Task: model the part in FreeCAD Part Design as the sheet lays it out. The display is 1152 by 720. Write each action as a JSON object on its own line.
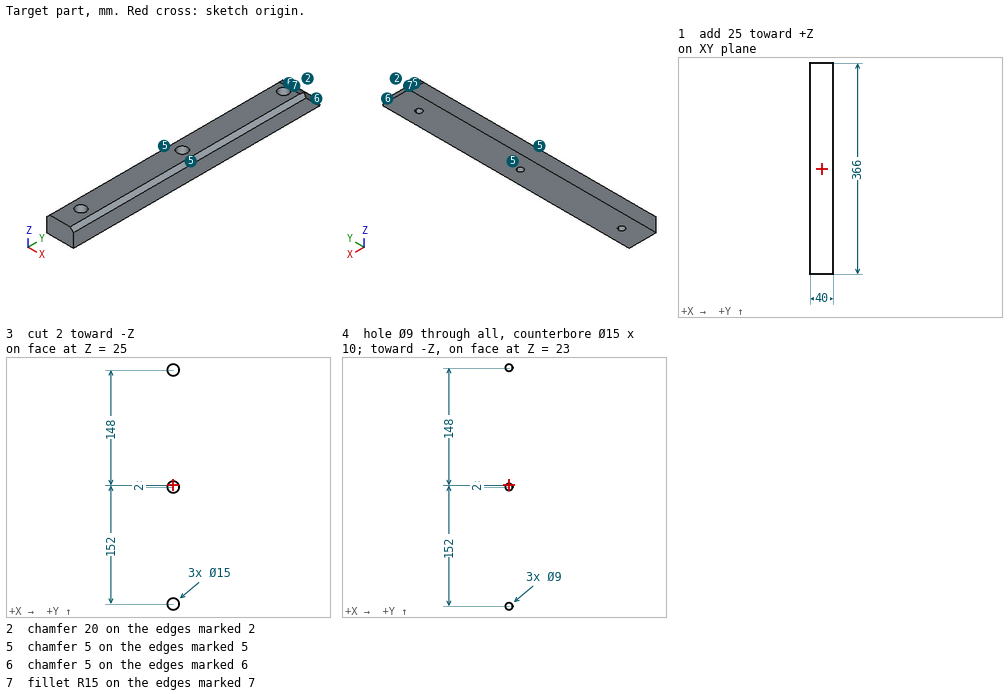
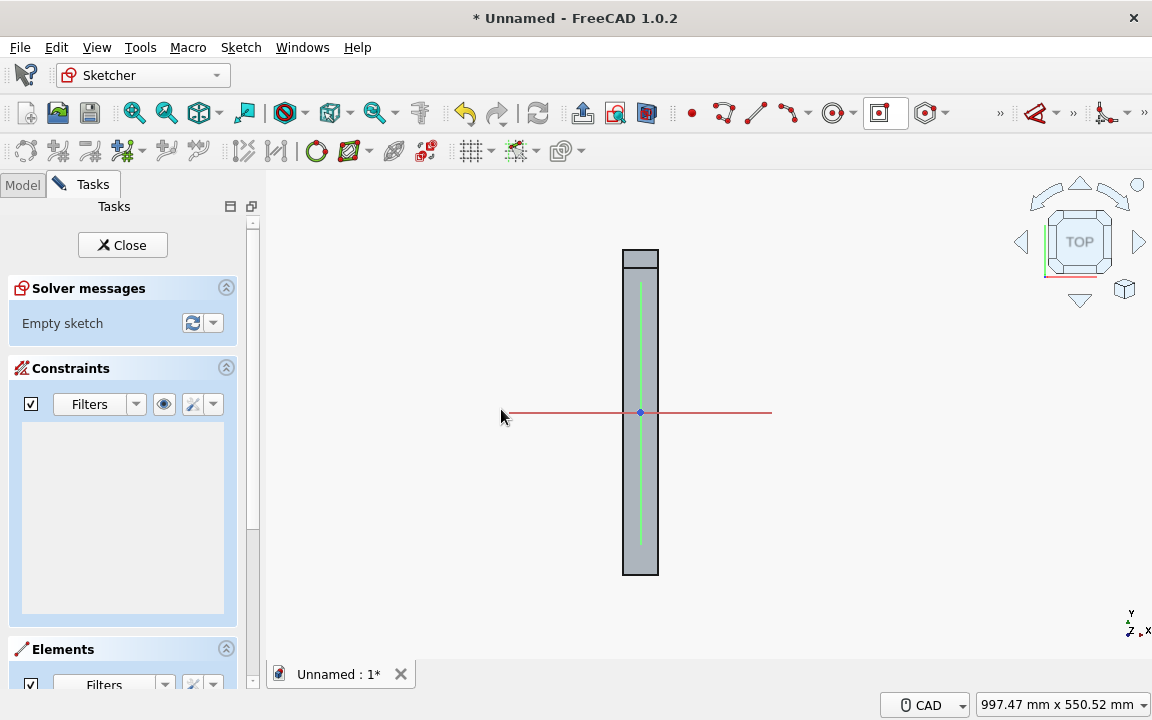
{"action": "left_click", "coordinate": [834, 114]}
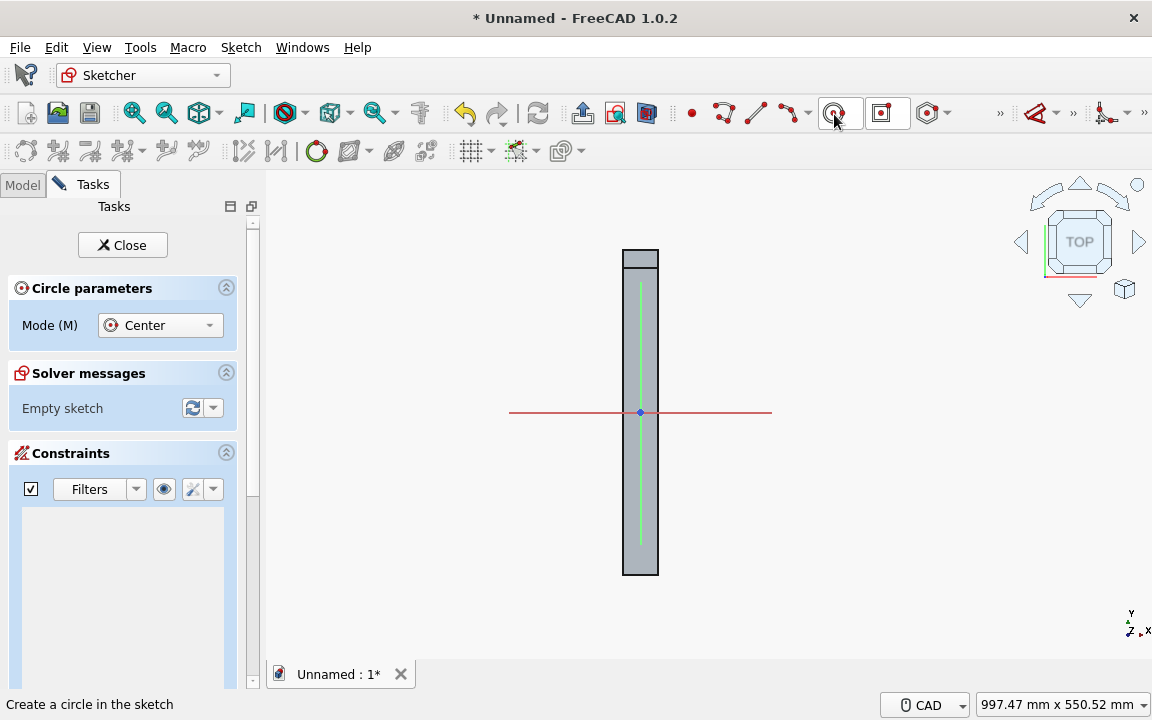
{"action": "scroll", "coordinate": [641, 548], "scroll_direction": "up", "scroll_amount": 7}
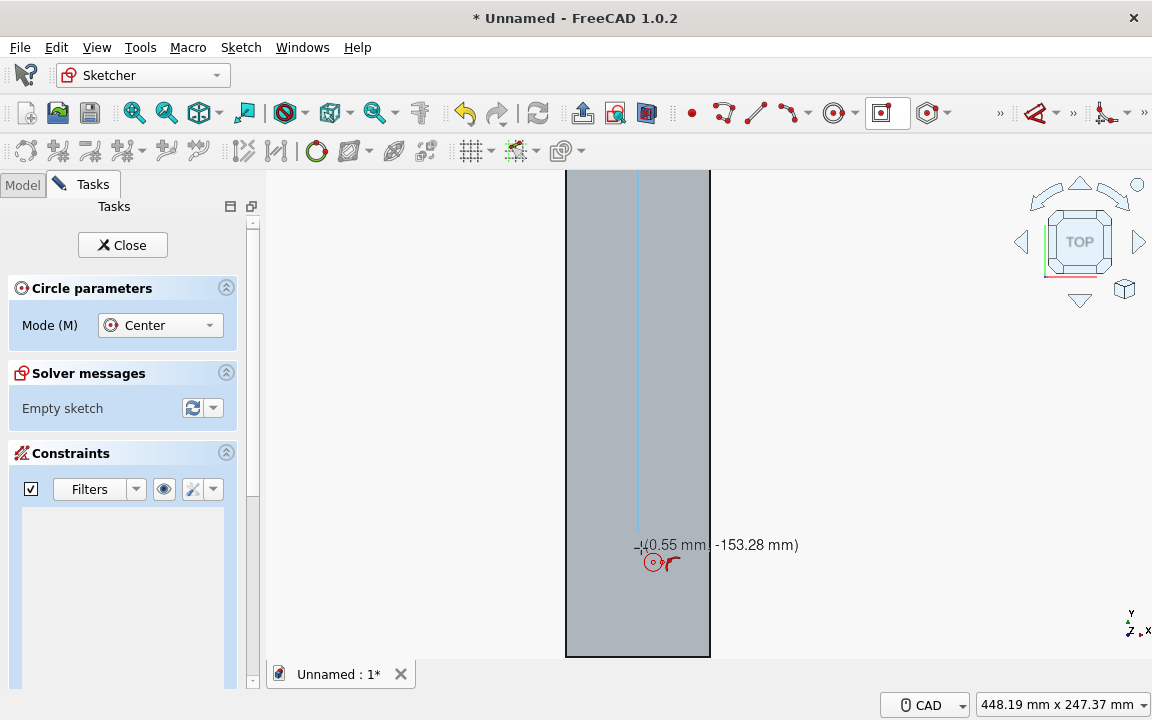
{"action": "scroll", "coordinate": [641, 549], "scroll_direction": "down", "scroll_amount": 7}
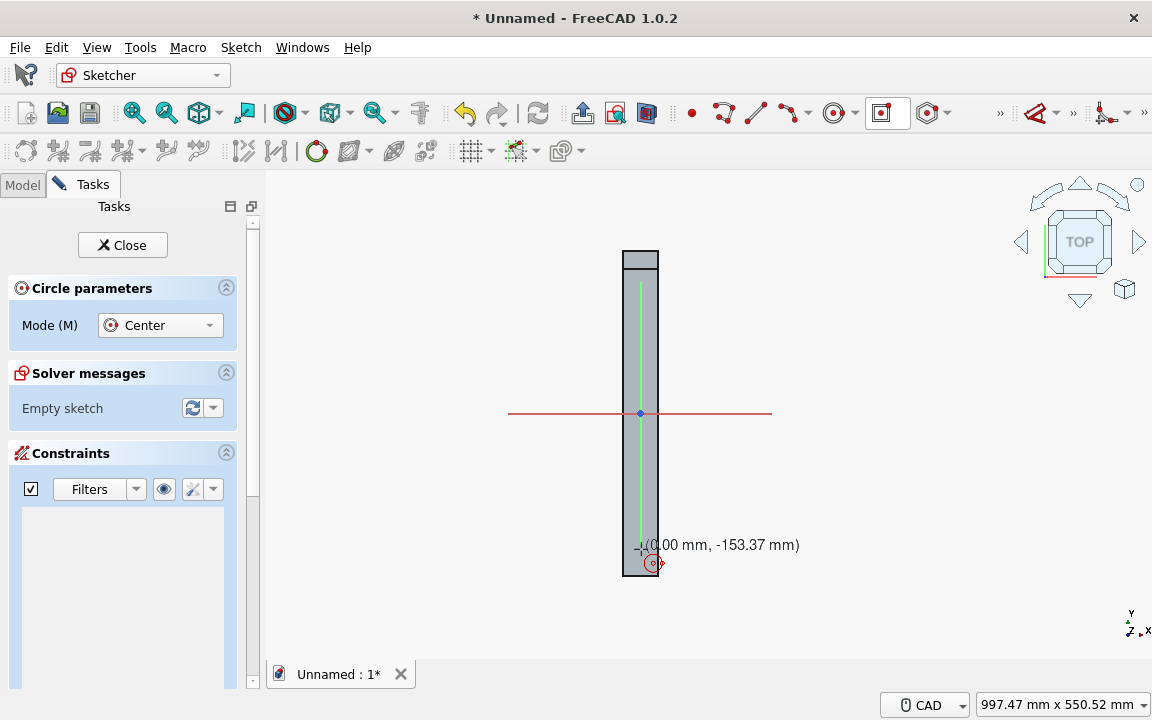
{"action": "left_click", "coordinate": [641, 549]}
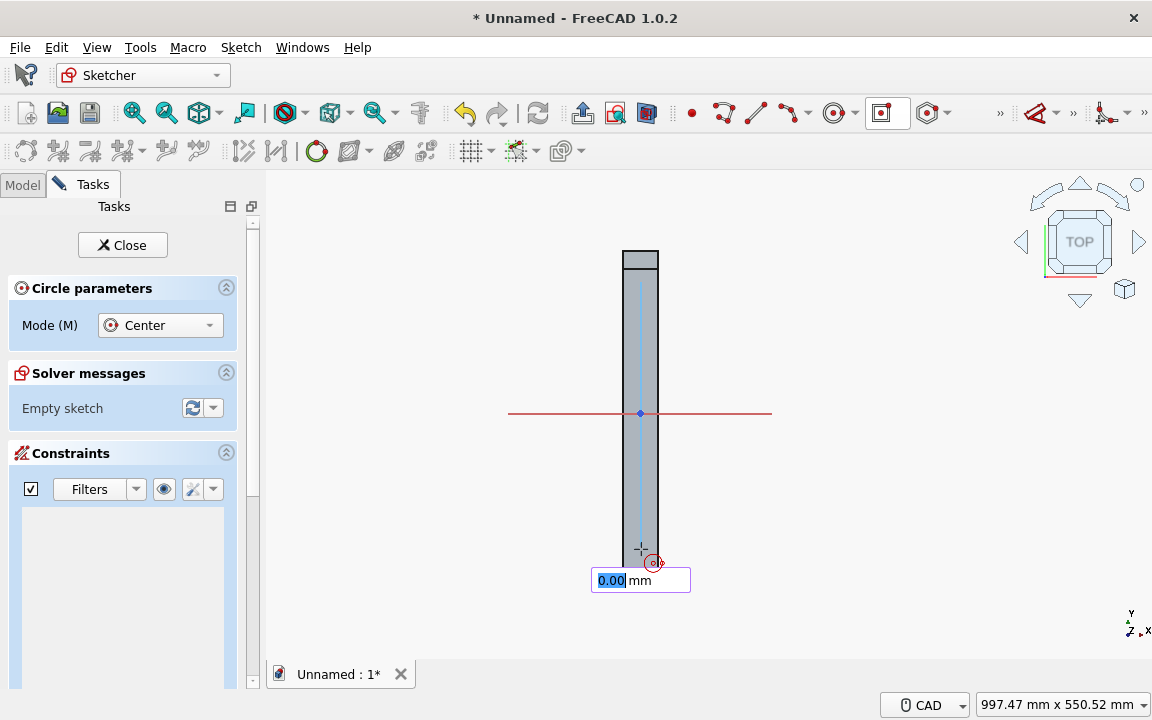
{"action": "scroll", "coordinate": [647, 546], "scroll_direction": "up", "scroll_amount": 5}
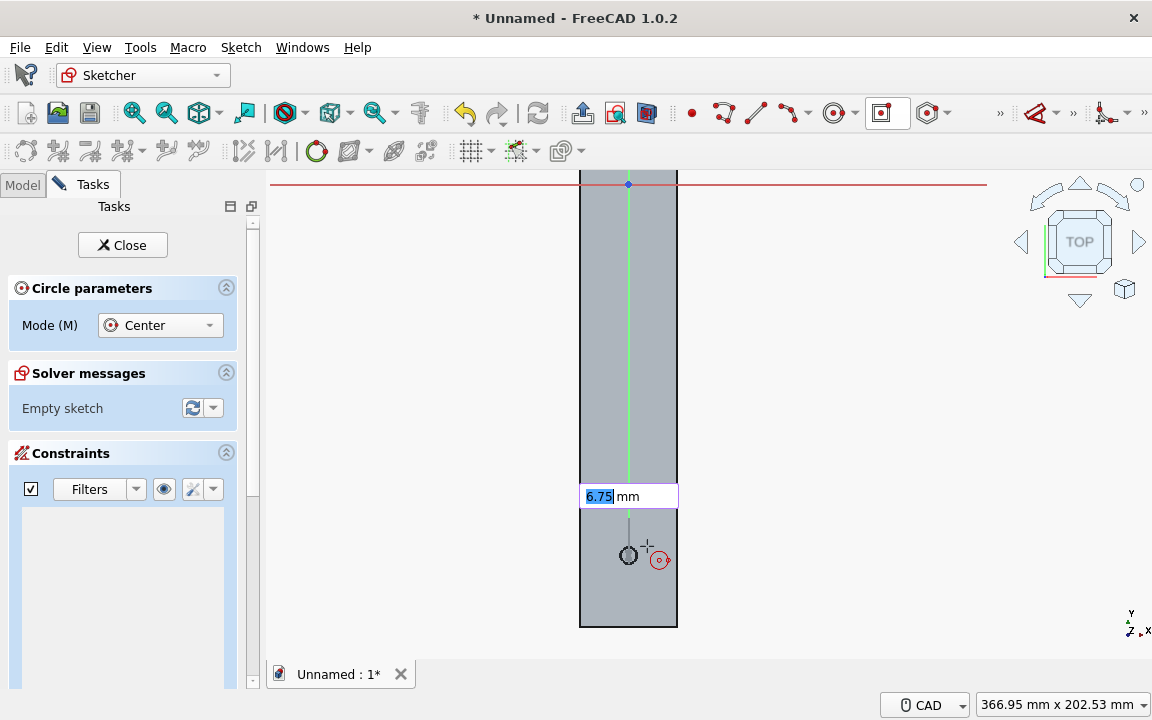
{"action": "left_click", "coordinate": [646, 546]}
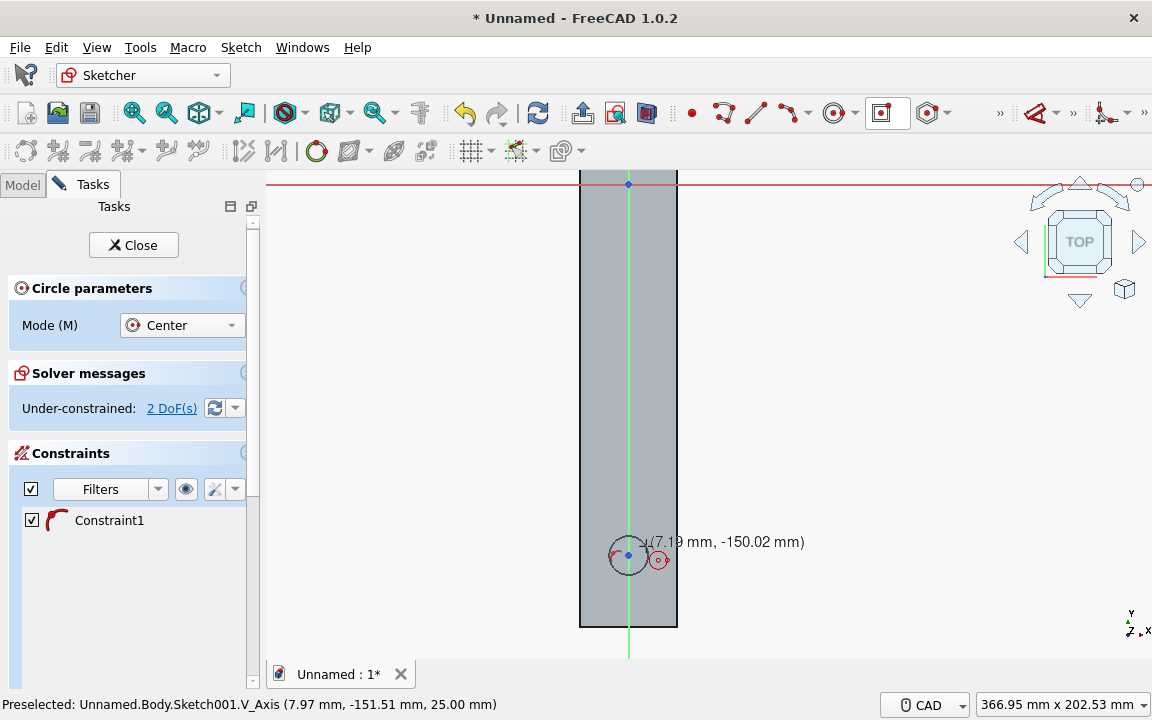
{"action": "scroll", "coordinate": [647, 545], "scroll_direction": "down", "scroll_amount": 5}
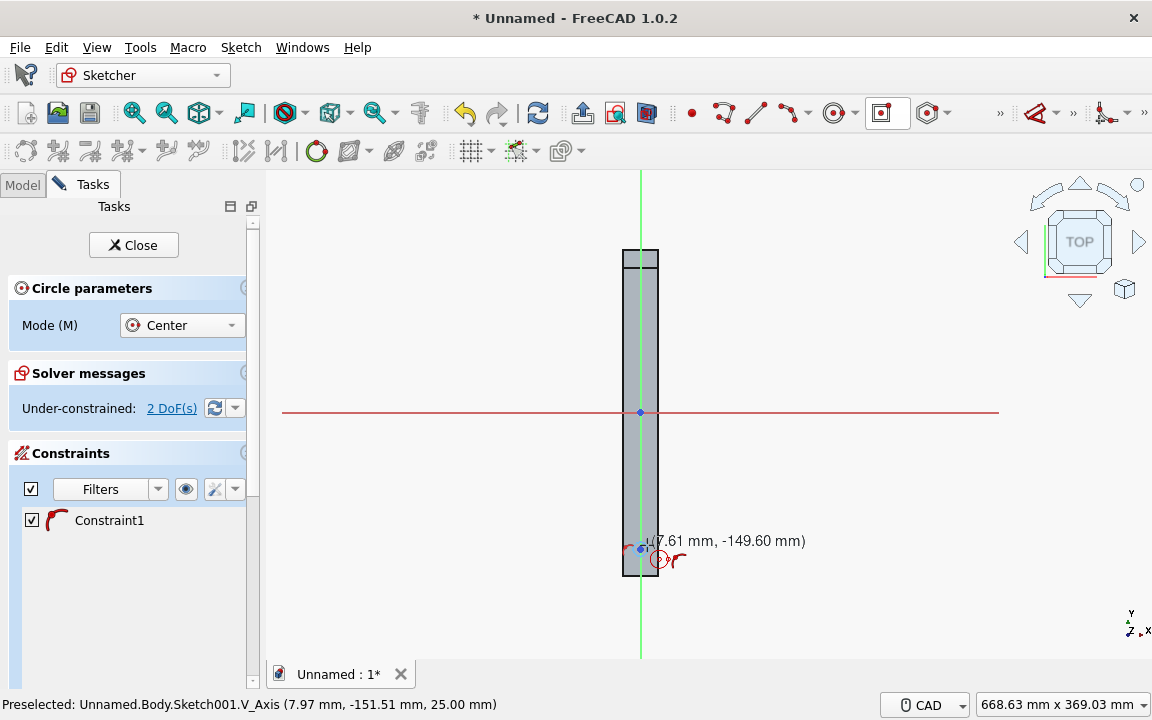
{"action": "scroll", "coordinate": [641, 415], "scroll_direction": "up", "scroll_amount": 11}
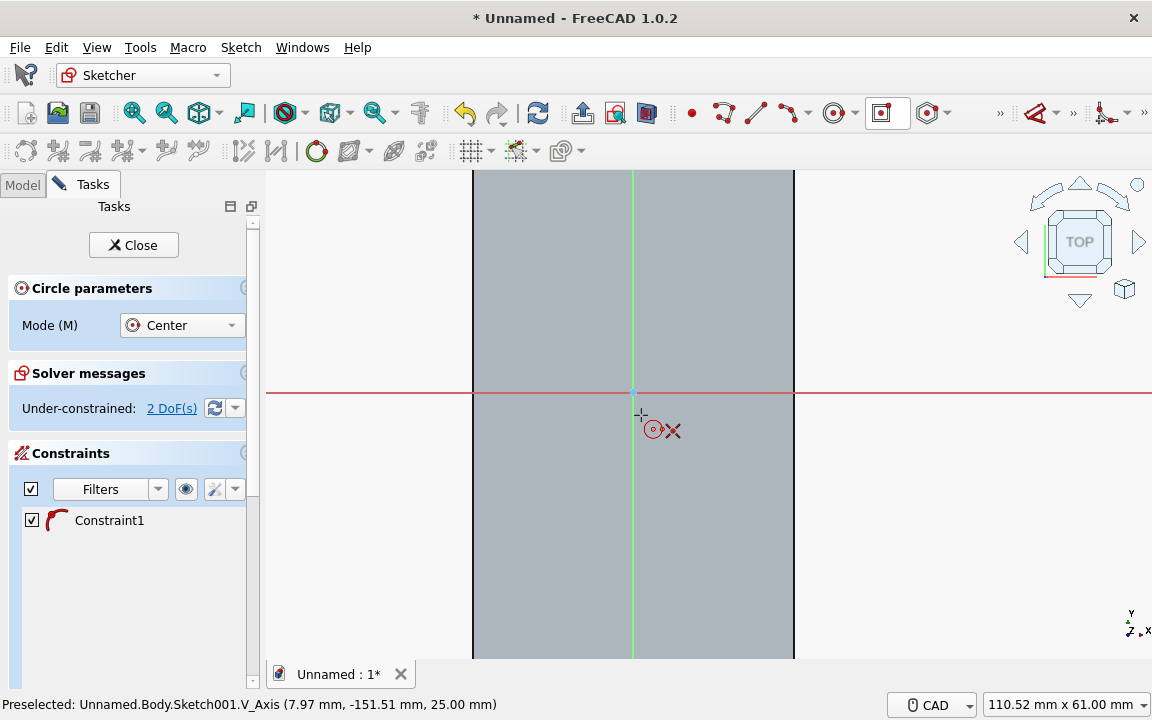
{"action": "left_click", "coordinate": [633, 409]}
{"action": "left_click", "coordinate": [676, 366]}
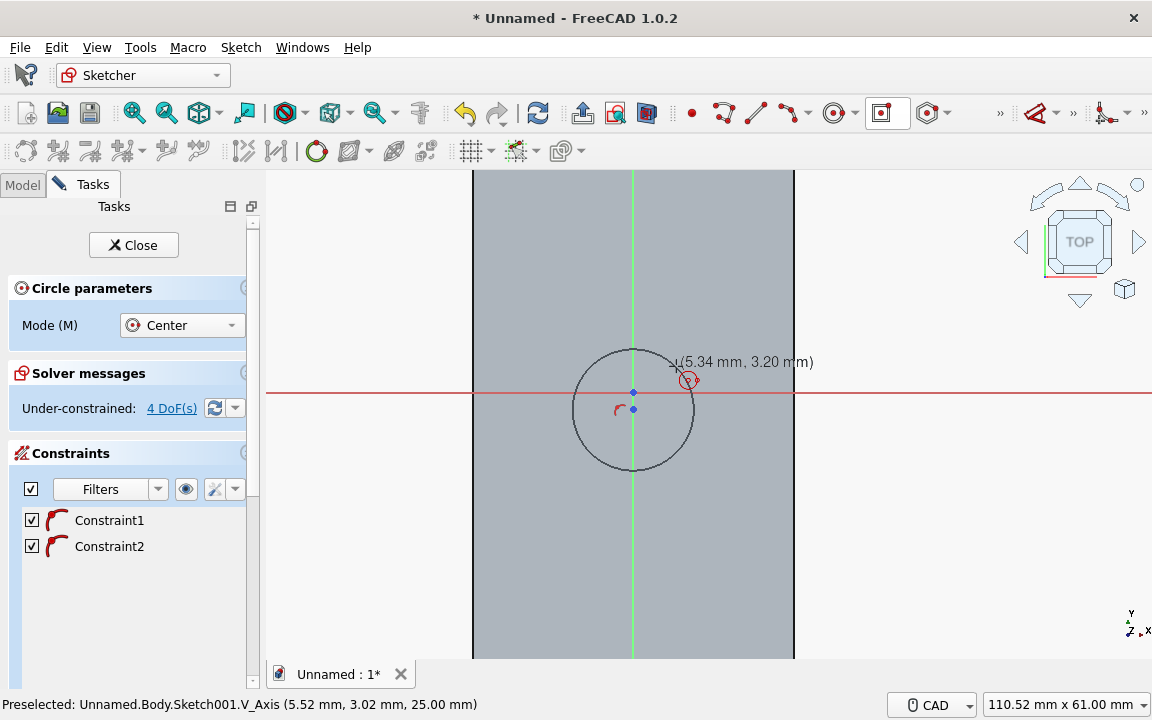
{"action": "scroll", "coordinate": [641, 415], "scroll_direction": "down", "scroll_amount": 11}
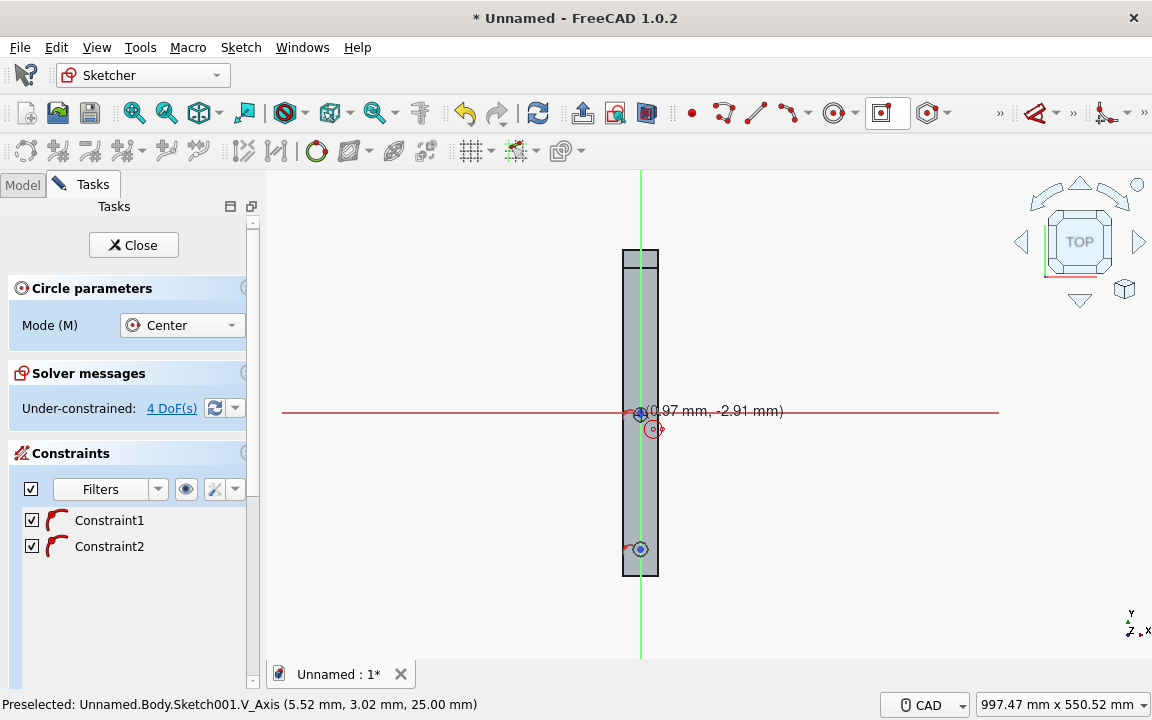
{"action": "scroll", "coordinate": [641, 282], "scroll_direction": "up", "scroll_amount": 7}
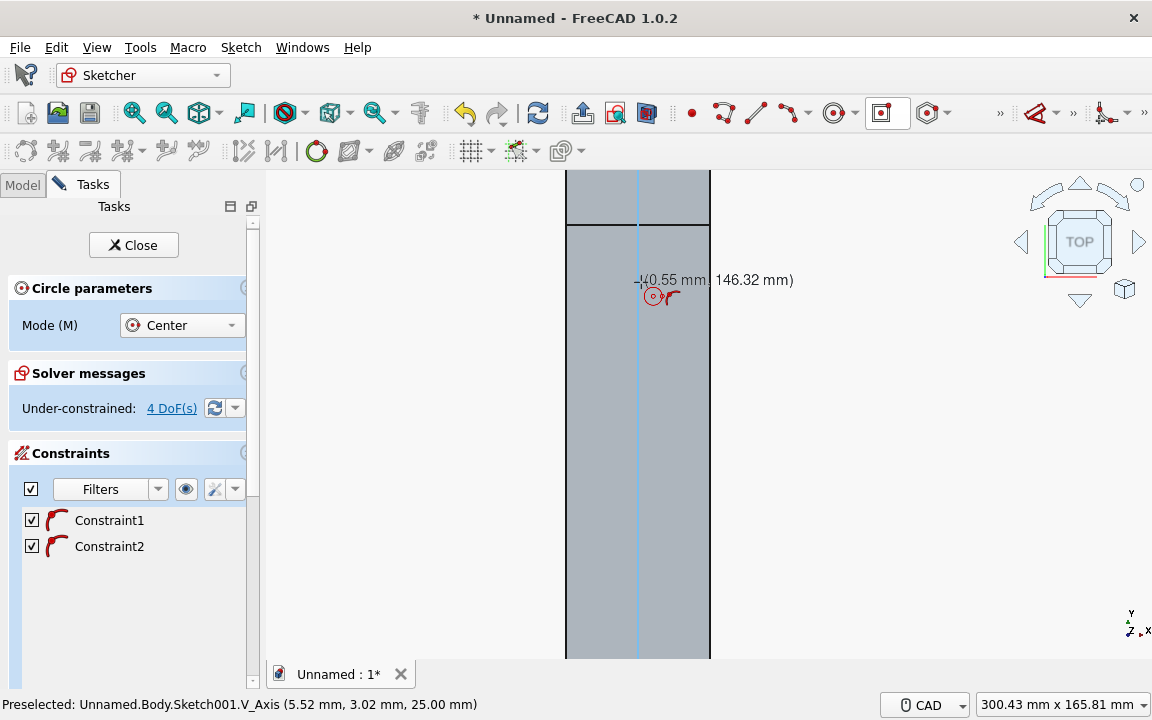
{"action": "scroll", "coordinate": [641, 282], "scroll_direction": "down", "scroll_amount": 7}